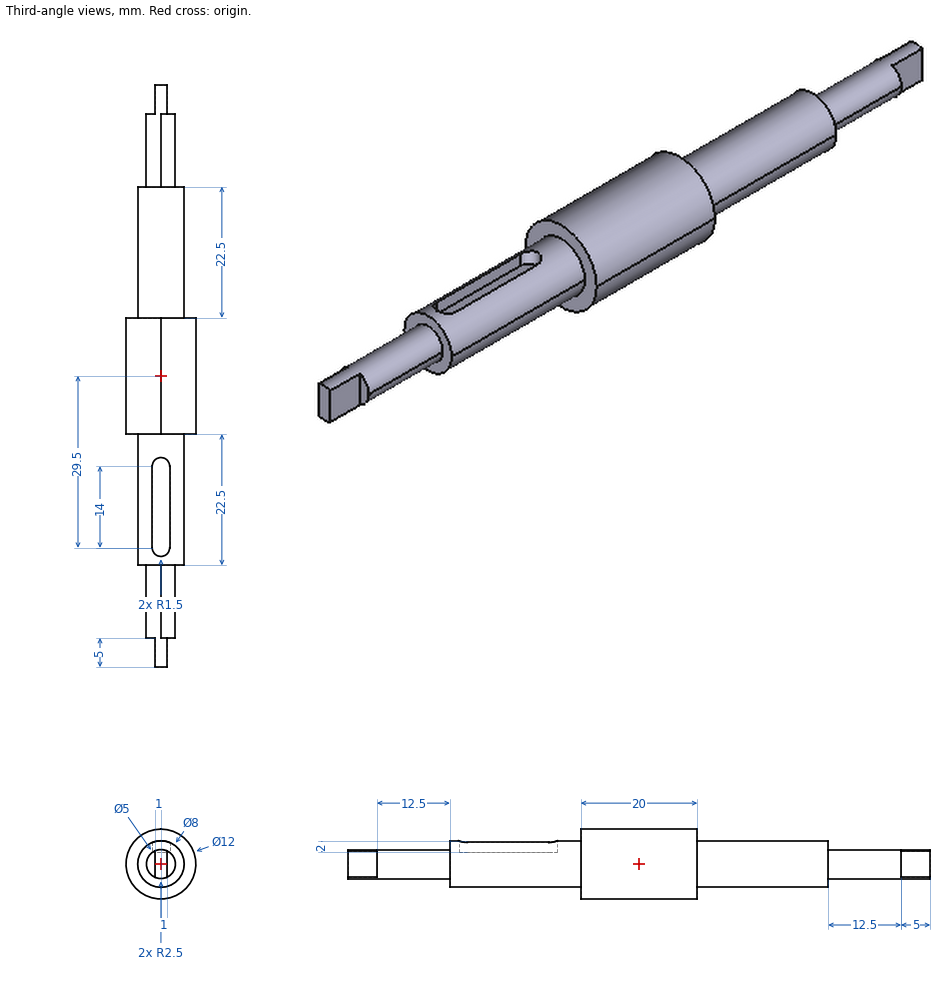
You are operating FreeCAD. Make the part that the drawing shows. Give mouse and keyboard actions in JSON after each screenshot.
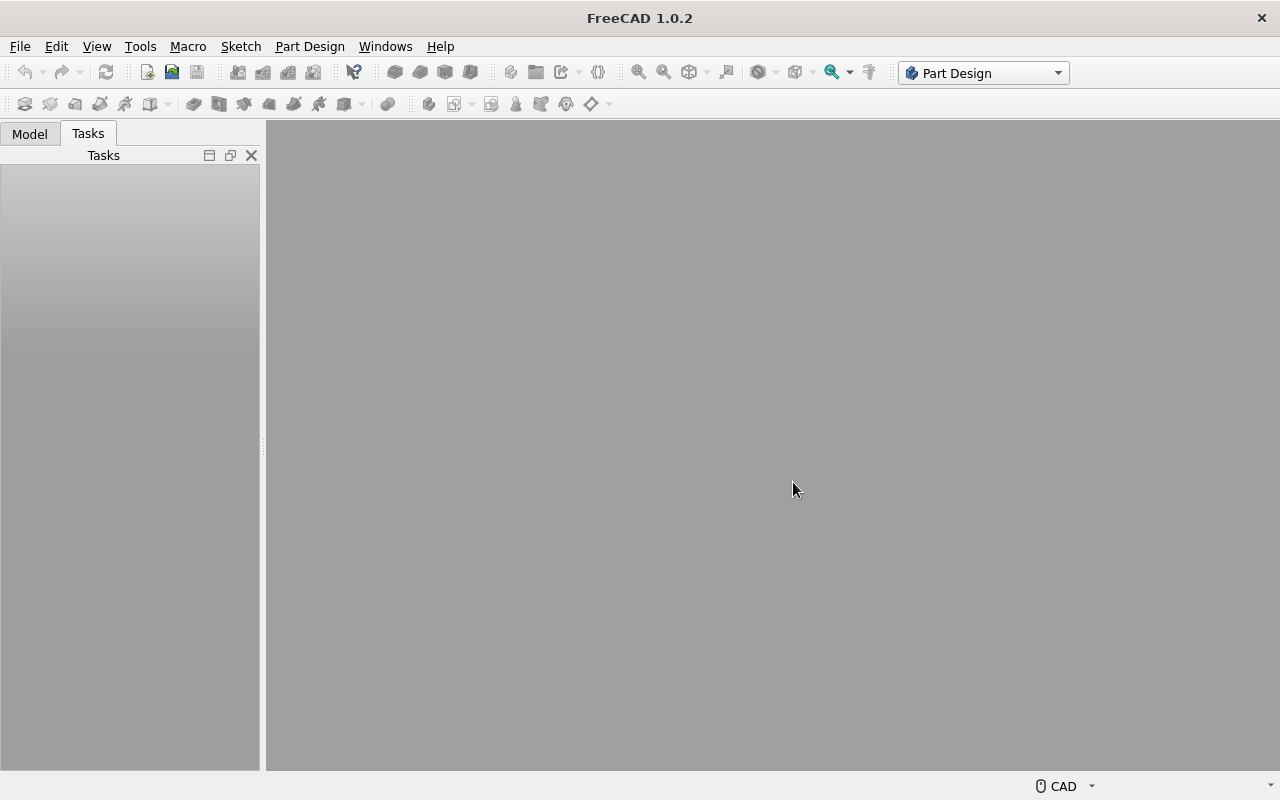
{"action": "key", "text": "ctrl+n"}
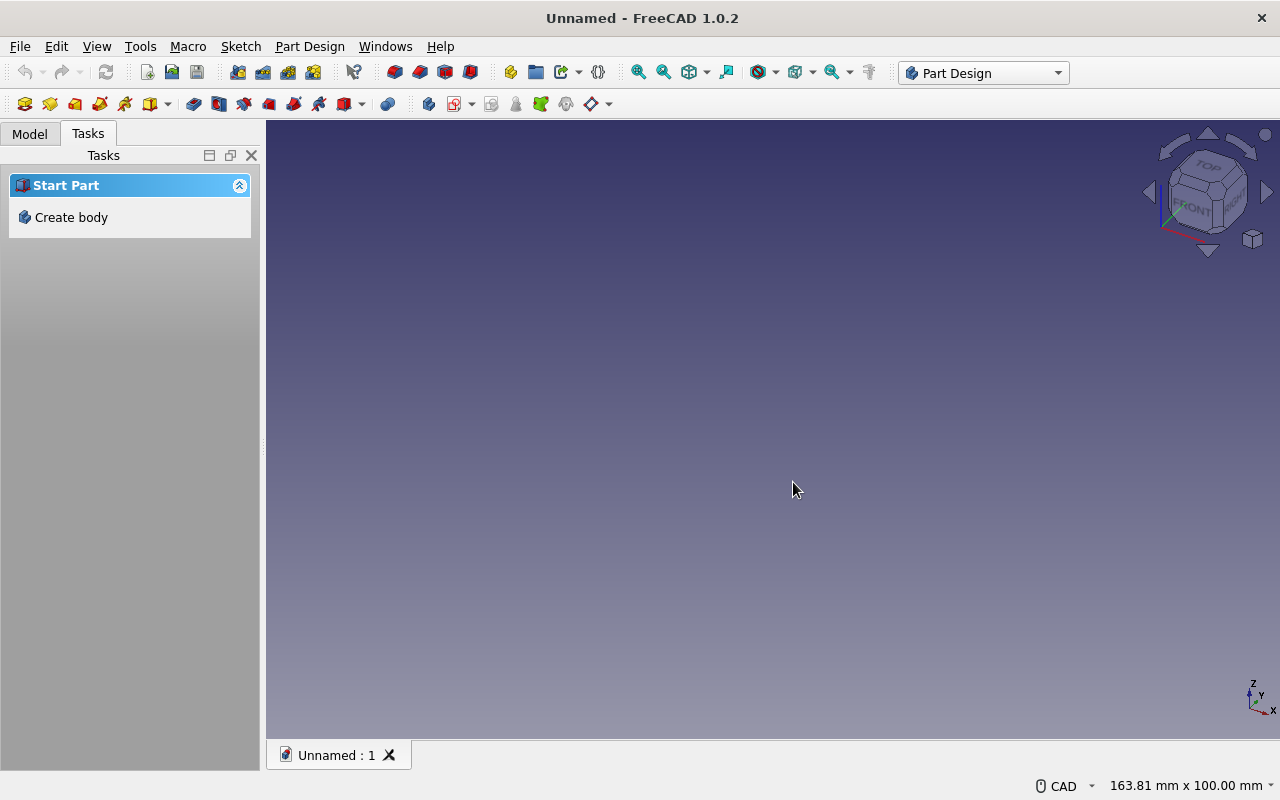
{"action": "left_click", "coordinate": [454, 104]}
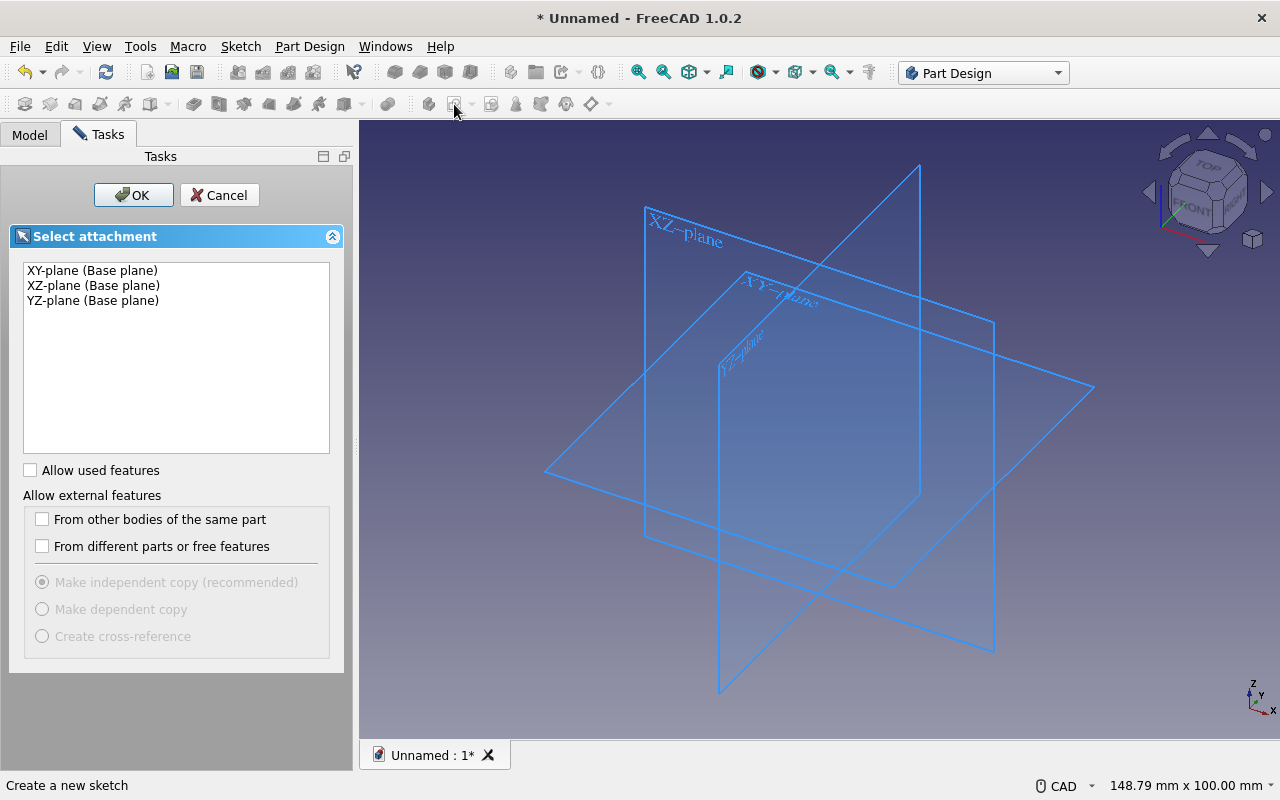
{"action": "left_click", "coordinate": [84, 286]}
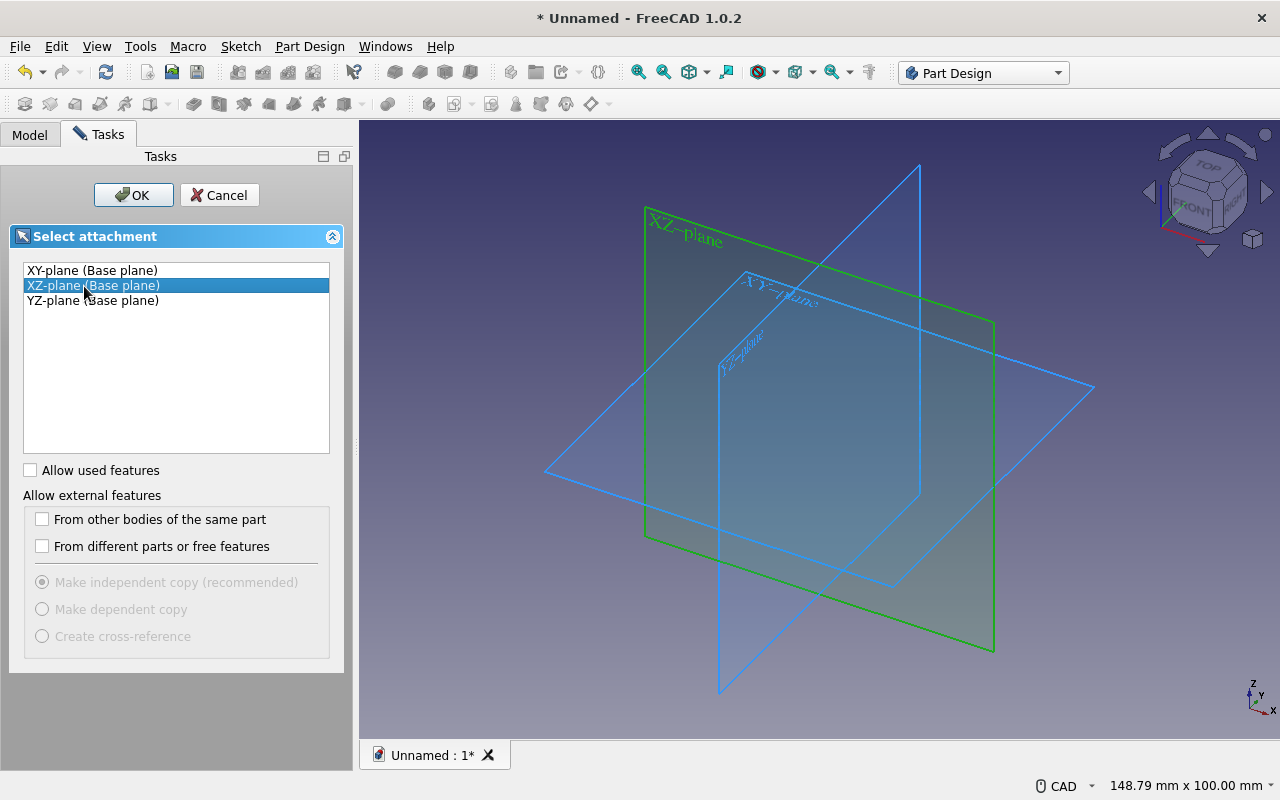
{"action": "left_click", "coordinate": [134, 195]}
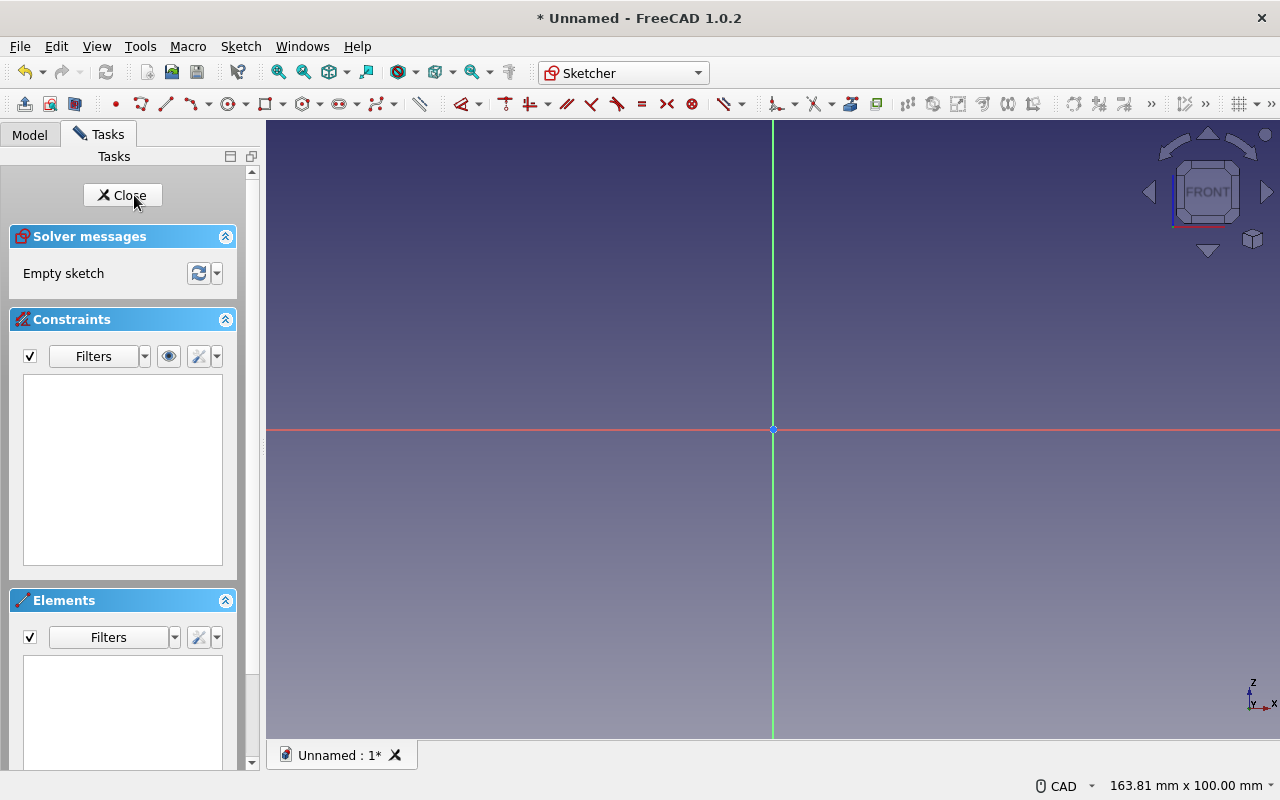
{"action": "scroll", "coordinate": [790, 430], "scroll_direction": "up", "scroll_amount": 8}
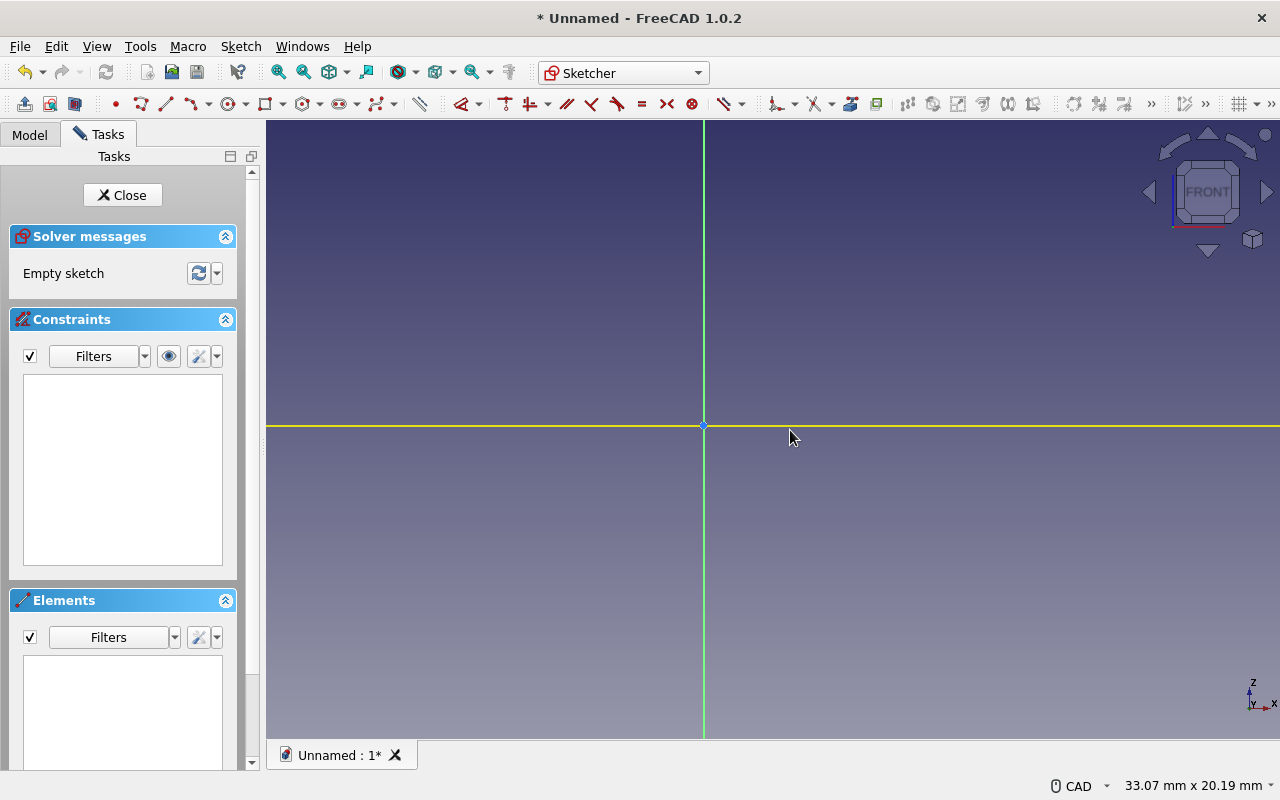
{"action": "key", "text": "g c"}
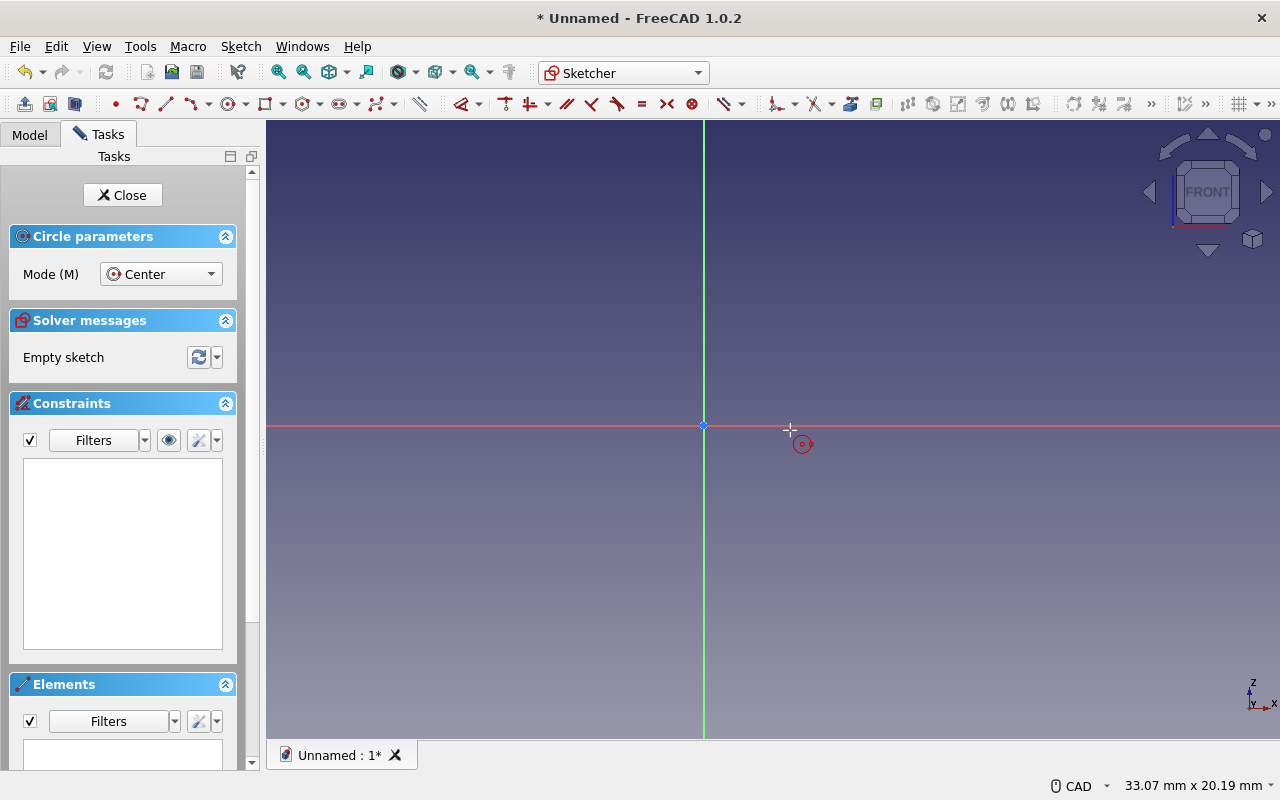
{"action": "left_click", "coordinate": [704, 426]}
{"action": "mouse_move", "coordinate": [834, 295]}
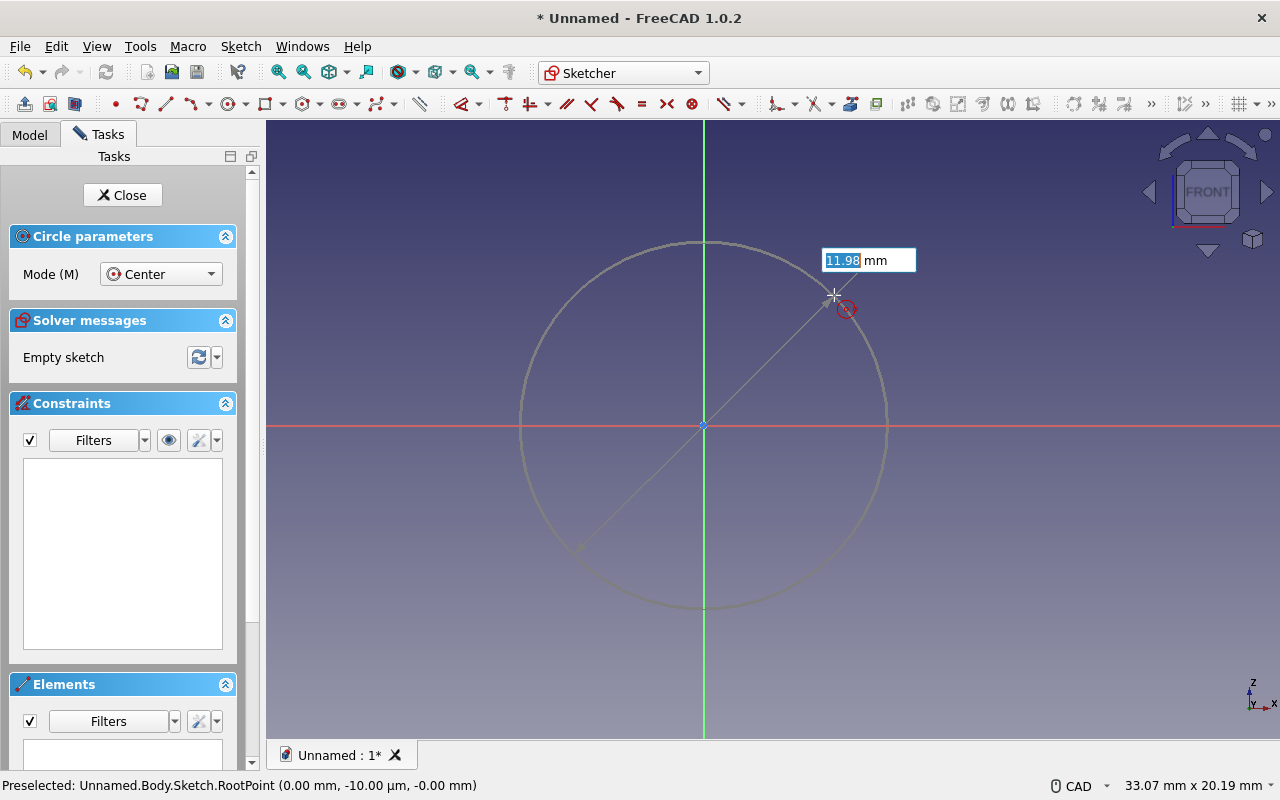
{"action": "type", "text": "12"}
{"action": "key", "text": "Return"}
{"action": "key", "text": "Escape"}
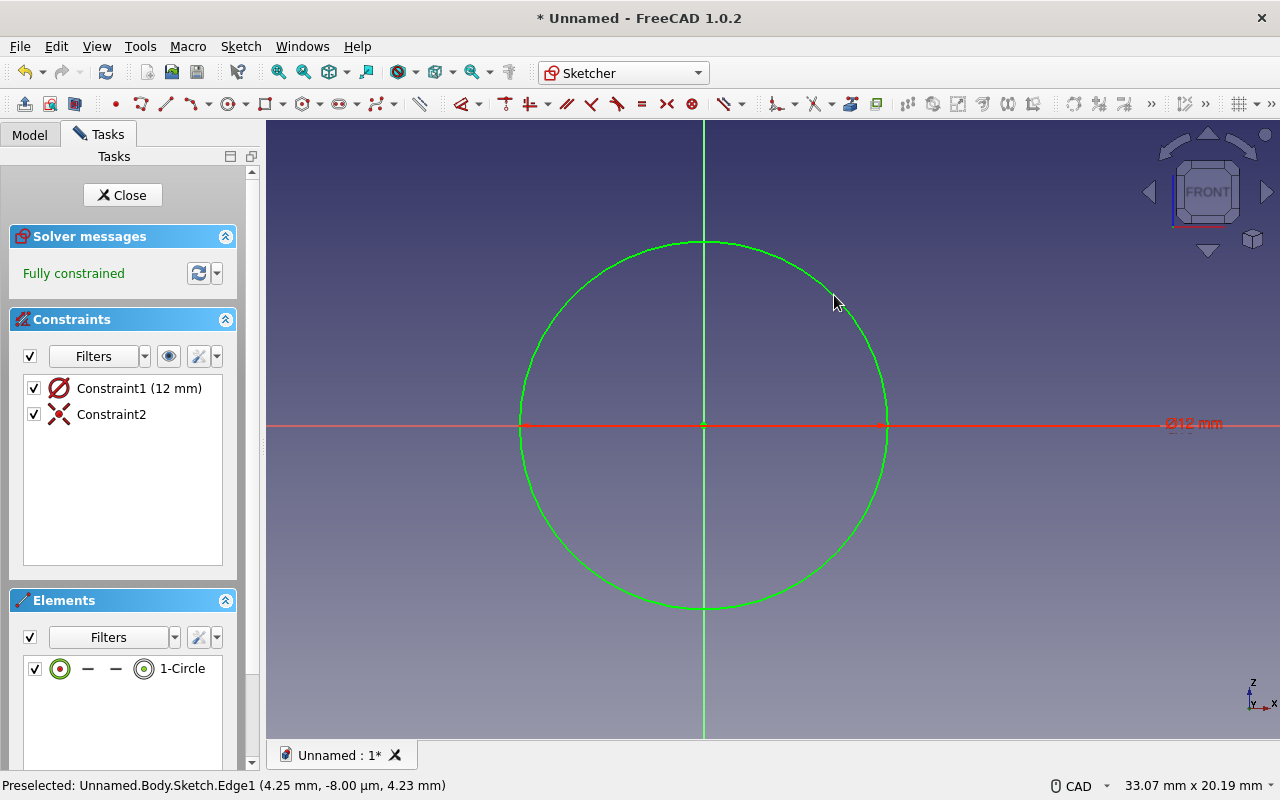
{"action": "left_click", "coordinate": [123, 195]}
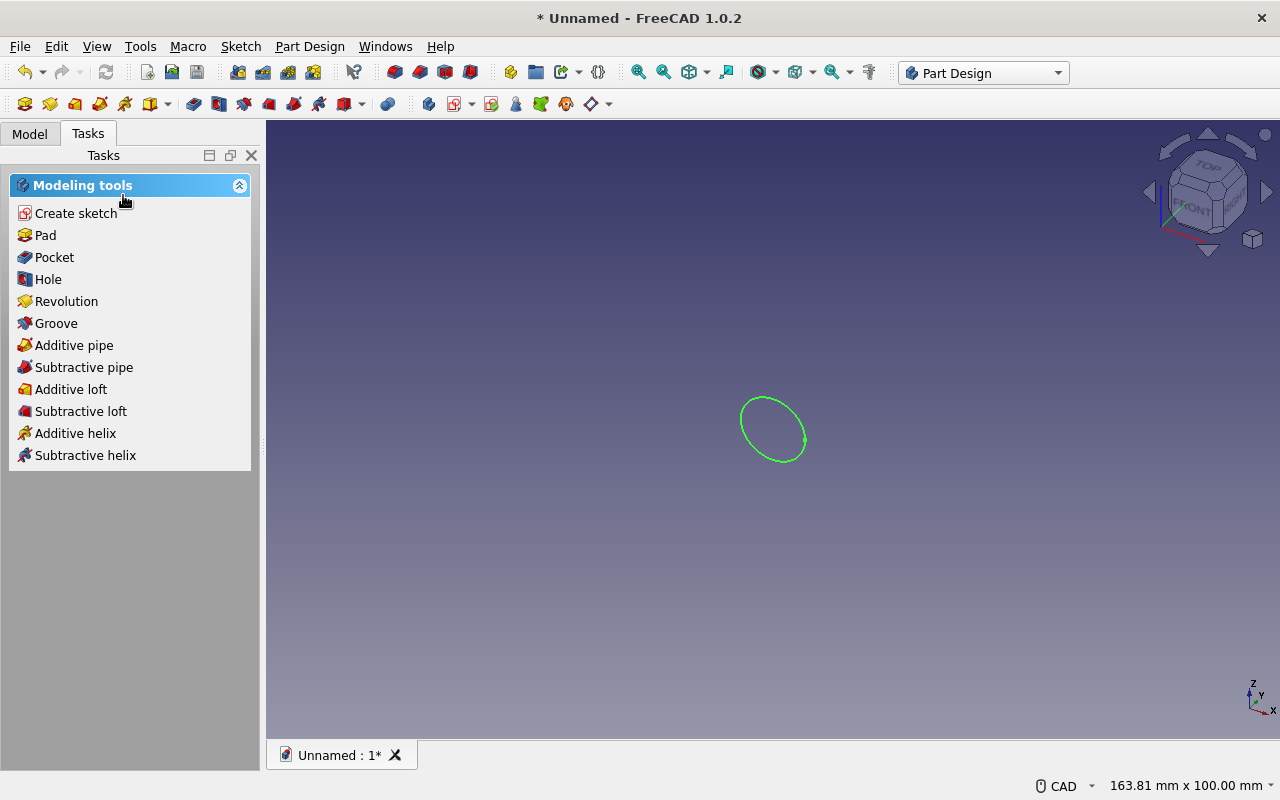
{"action": "left_click", "coordinate": [25, 104]}